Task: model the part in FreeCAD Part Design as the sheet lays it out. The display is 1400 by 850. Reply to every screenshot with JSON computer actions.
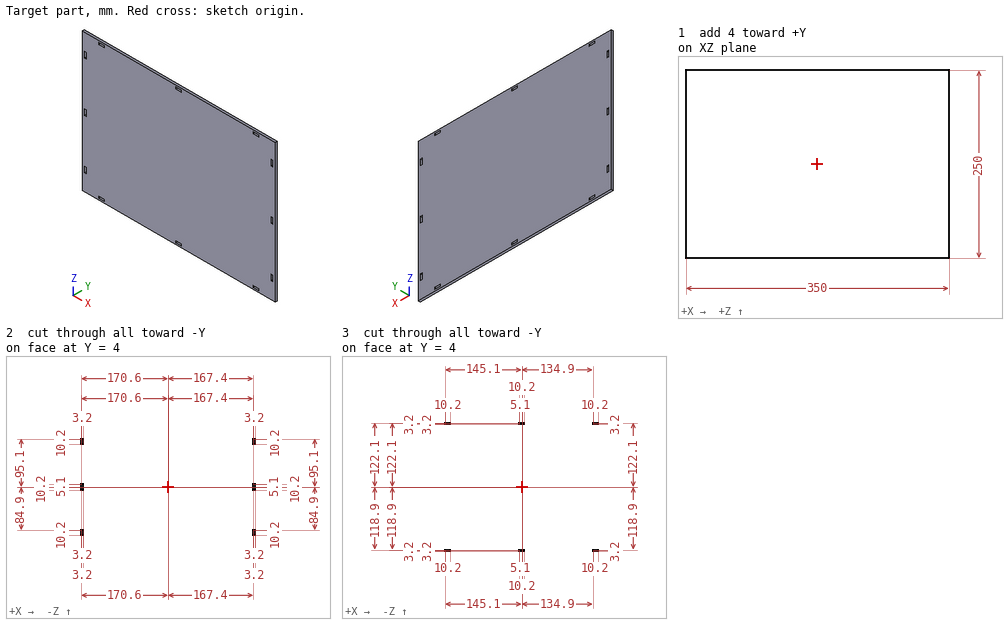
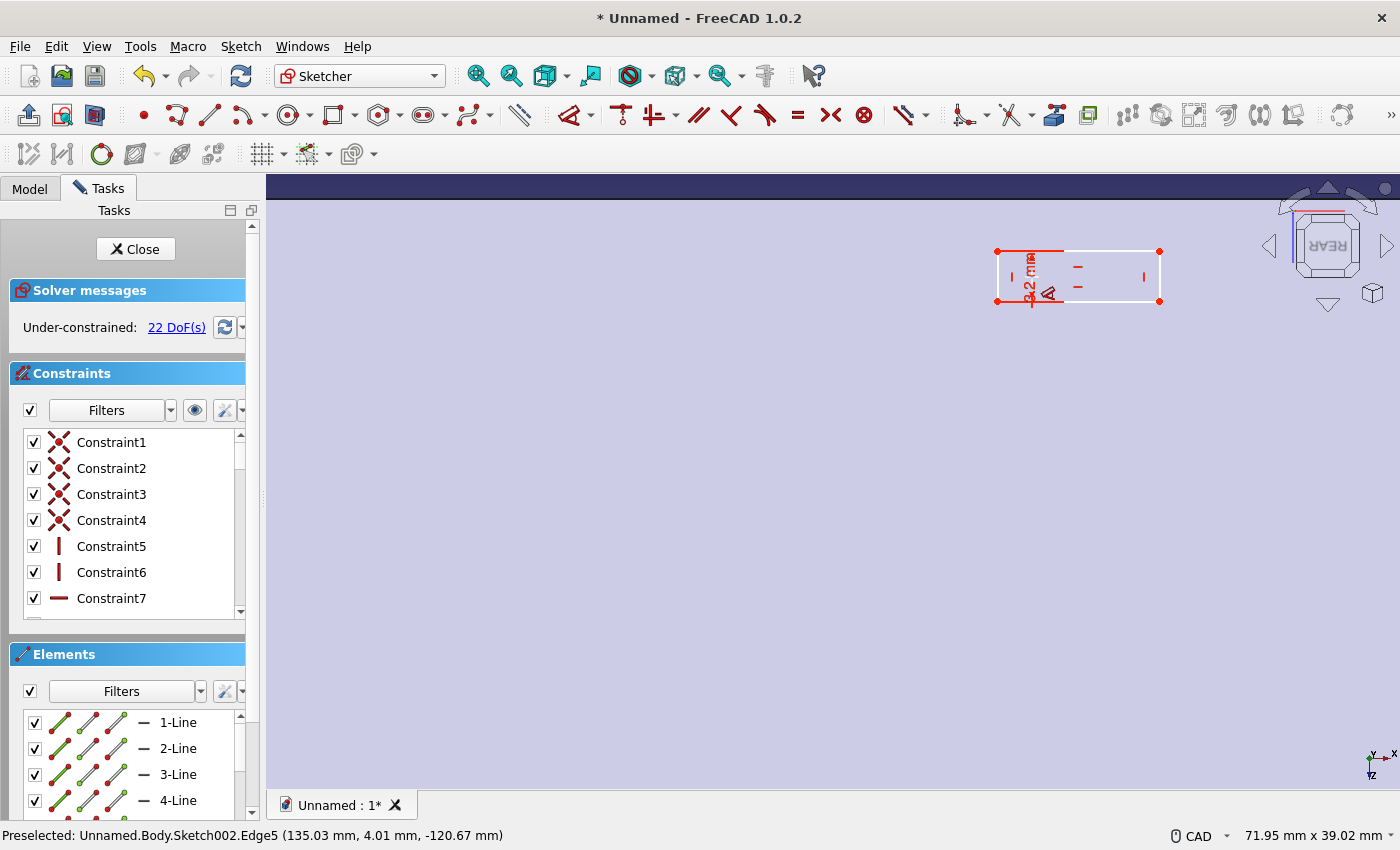
{"action": "scroll", "coordinate": [1001, 271], "scroll_direction": "down", "scroll_amount": 11}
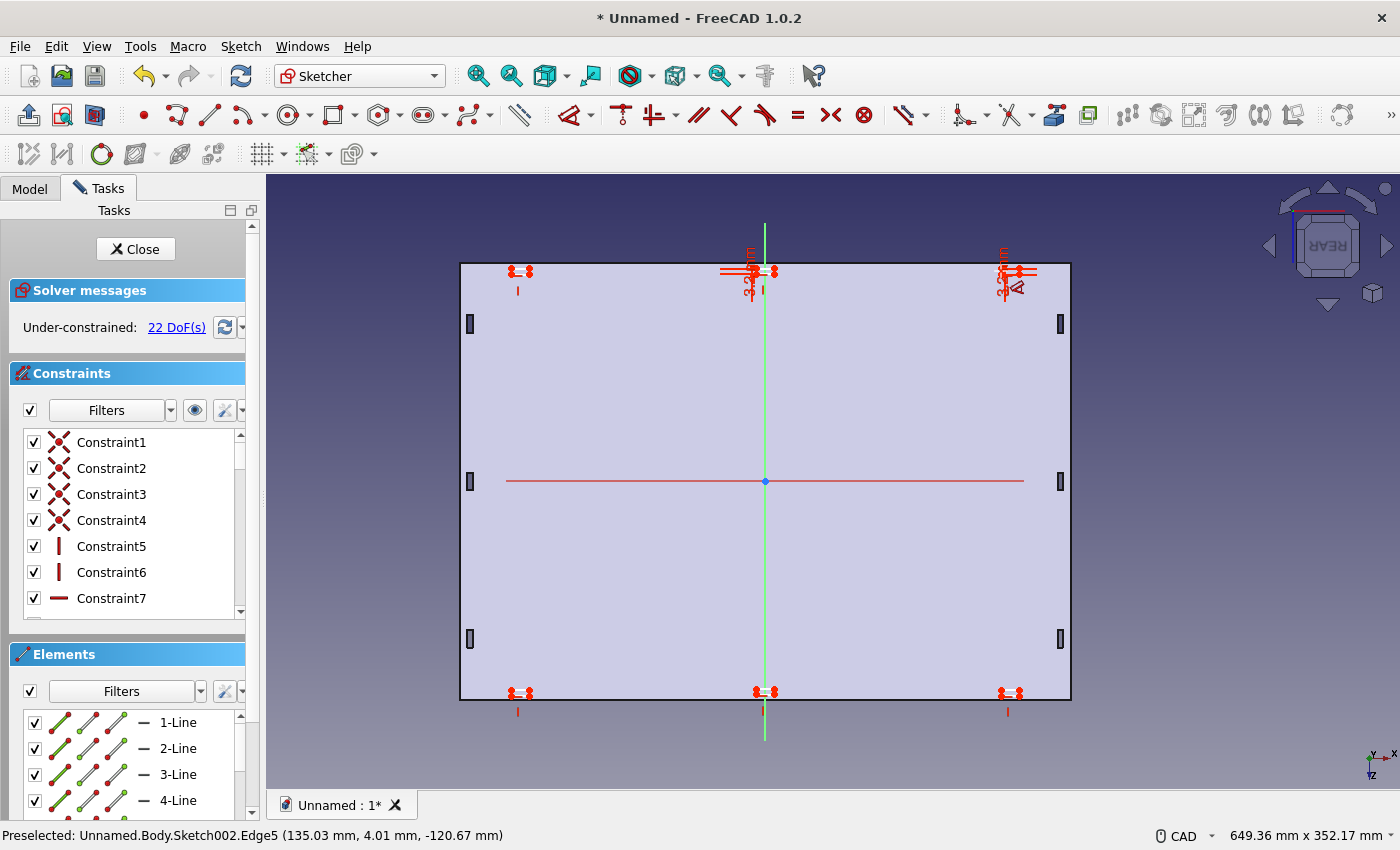
{"action": "scroll", "coordinate": [512, 271], "scroll_direction": "up", "scroll_amount": 11}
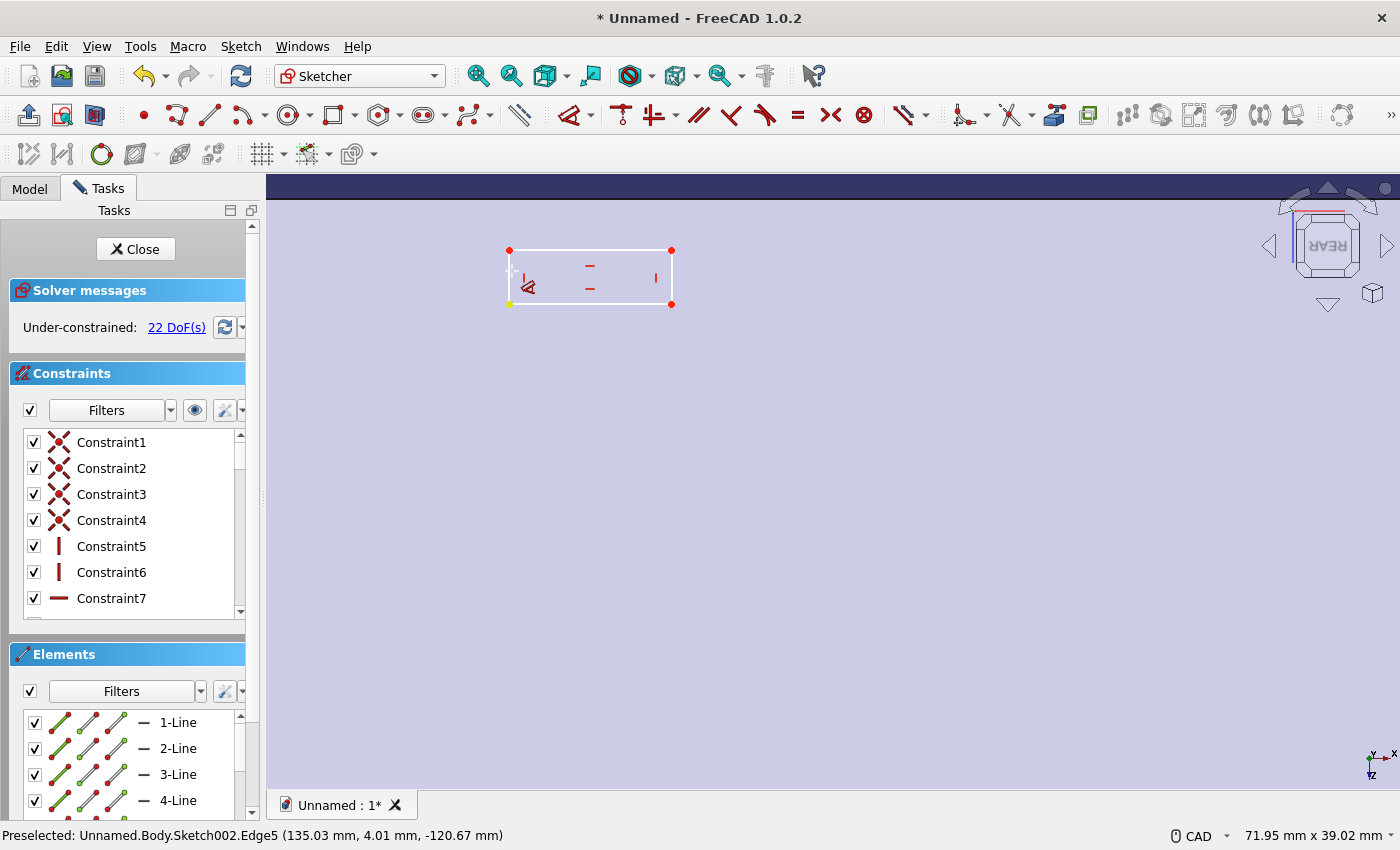
{"action": "left_click", "coordinate": [509, 266]}
{"action": "left_click", "coordinate": [475, 277]}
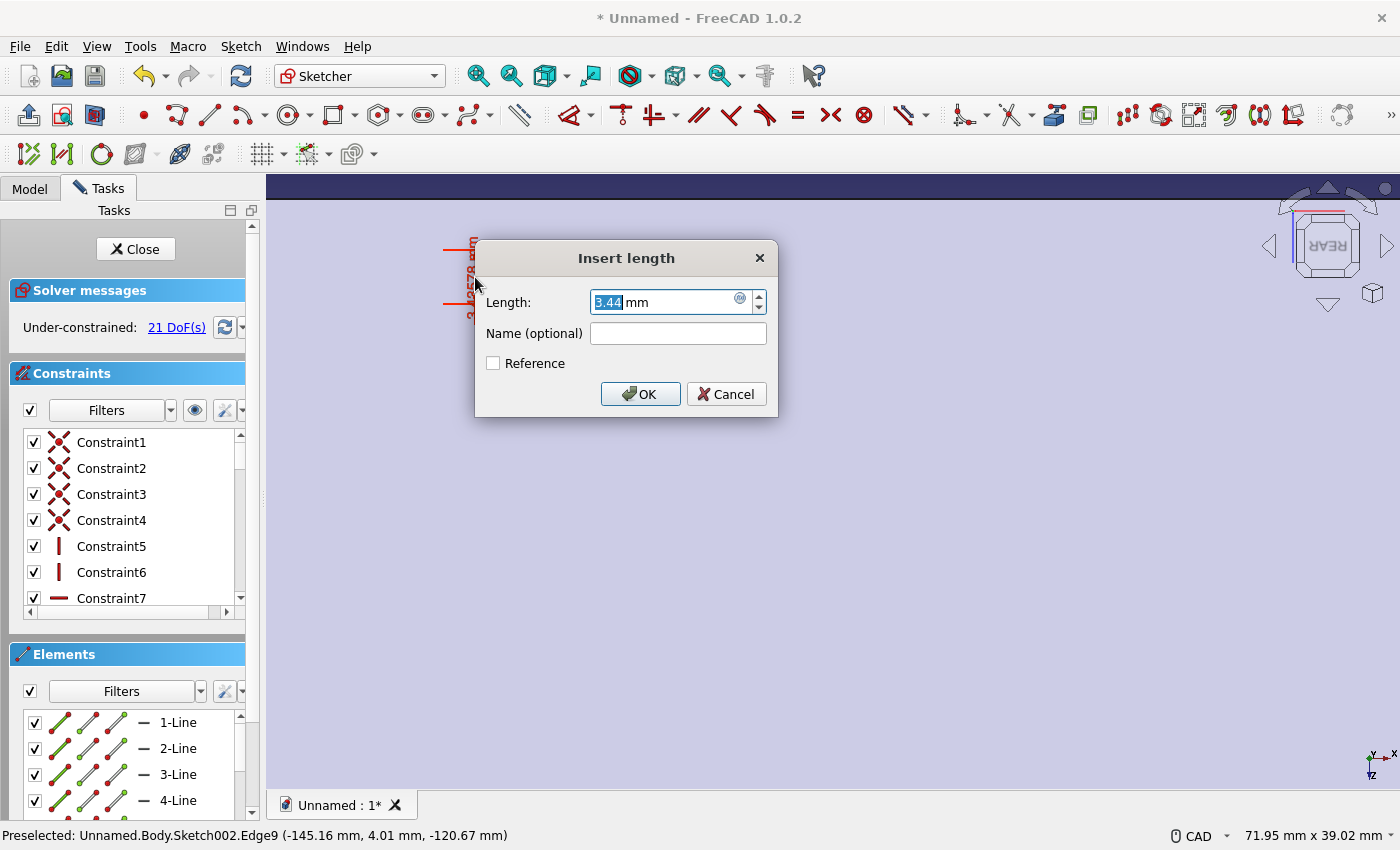
{"action": "type", "text": "3.2"}
{"action": "key", "text": "Return"}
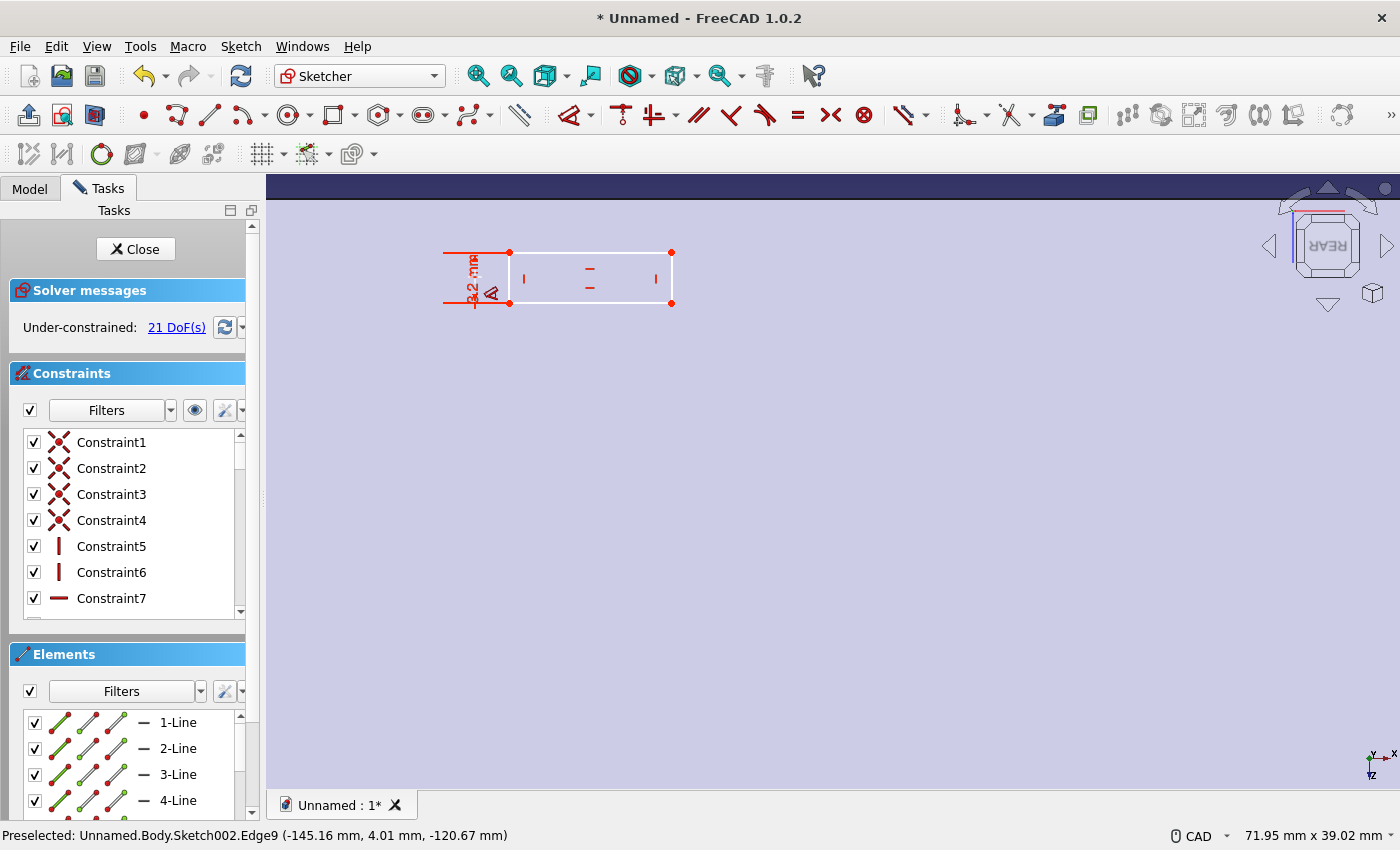
{"action": "scroll", "coordinate": [511, 271], "scroll_direction": "down", "scroll_amount": 11}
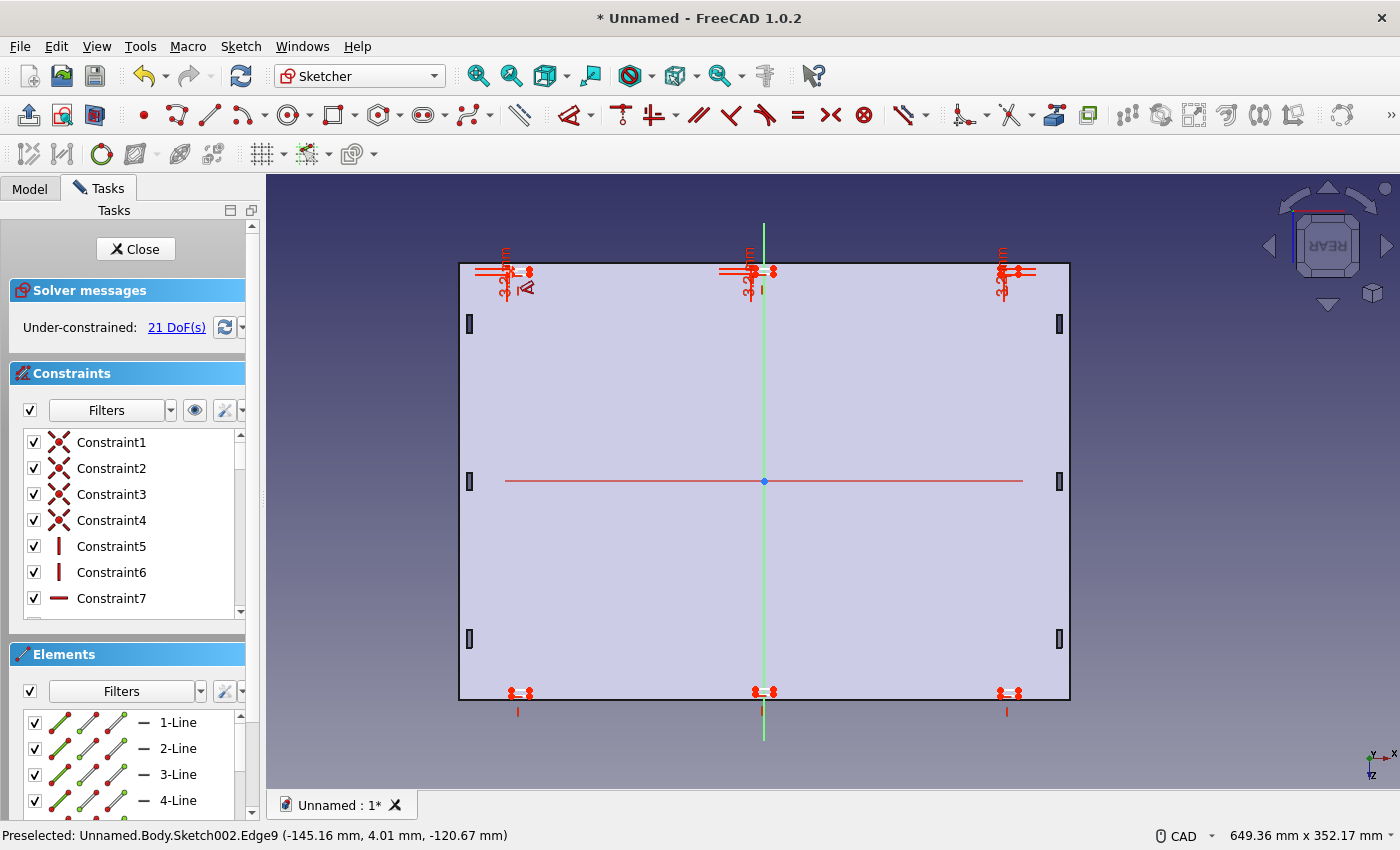
{"action": "scroll", "coordinate": [511, 692], "scroll_direction": "up", "scroll_amount": 11}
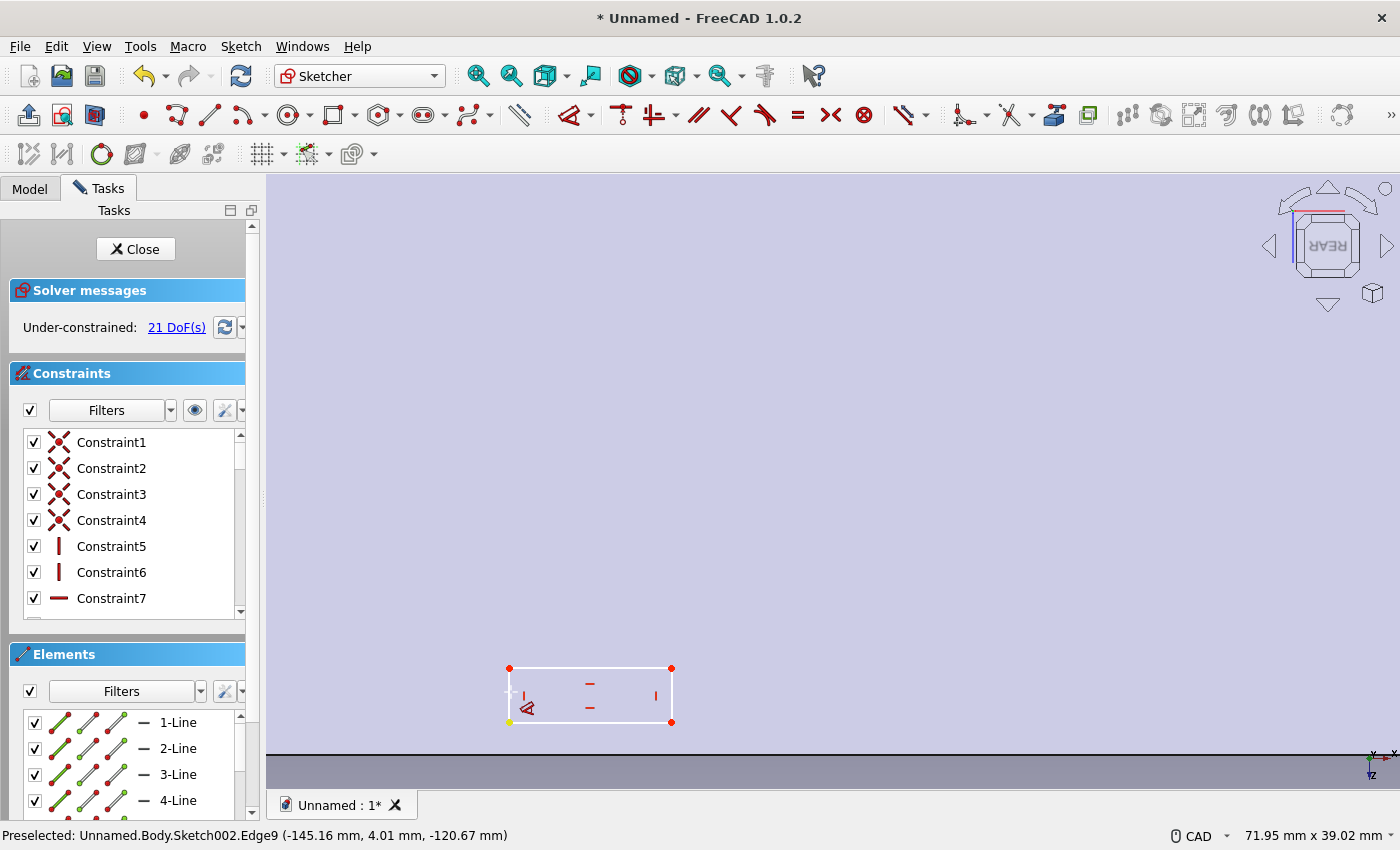
{"action": "left_click", "coordinate": [509, 685]}
{"action": "left_click", "coordinate": [475, 695]}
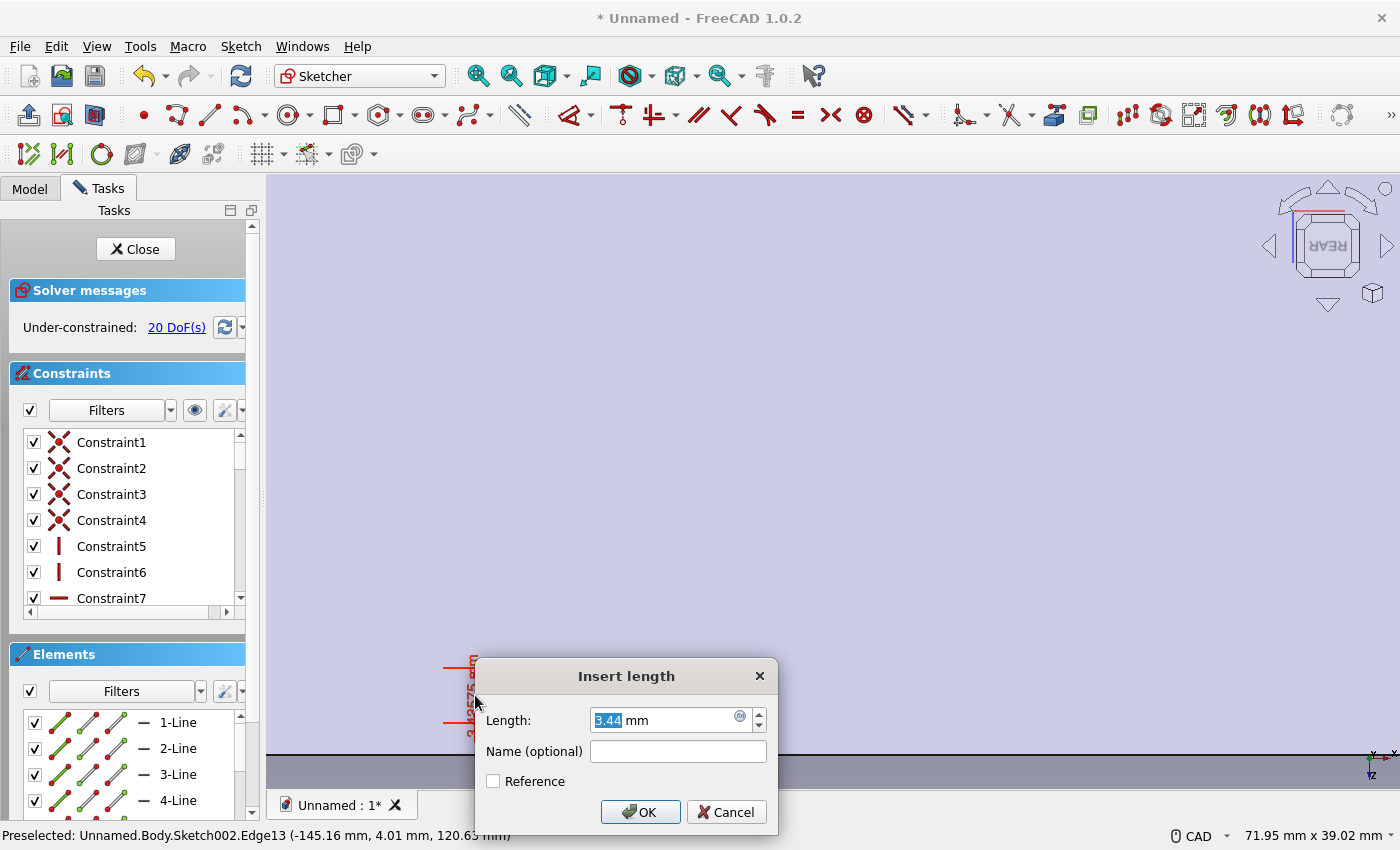
{"action": "type", "text": "3.2"}
{"action": "key", "text": "Return"}